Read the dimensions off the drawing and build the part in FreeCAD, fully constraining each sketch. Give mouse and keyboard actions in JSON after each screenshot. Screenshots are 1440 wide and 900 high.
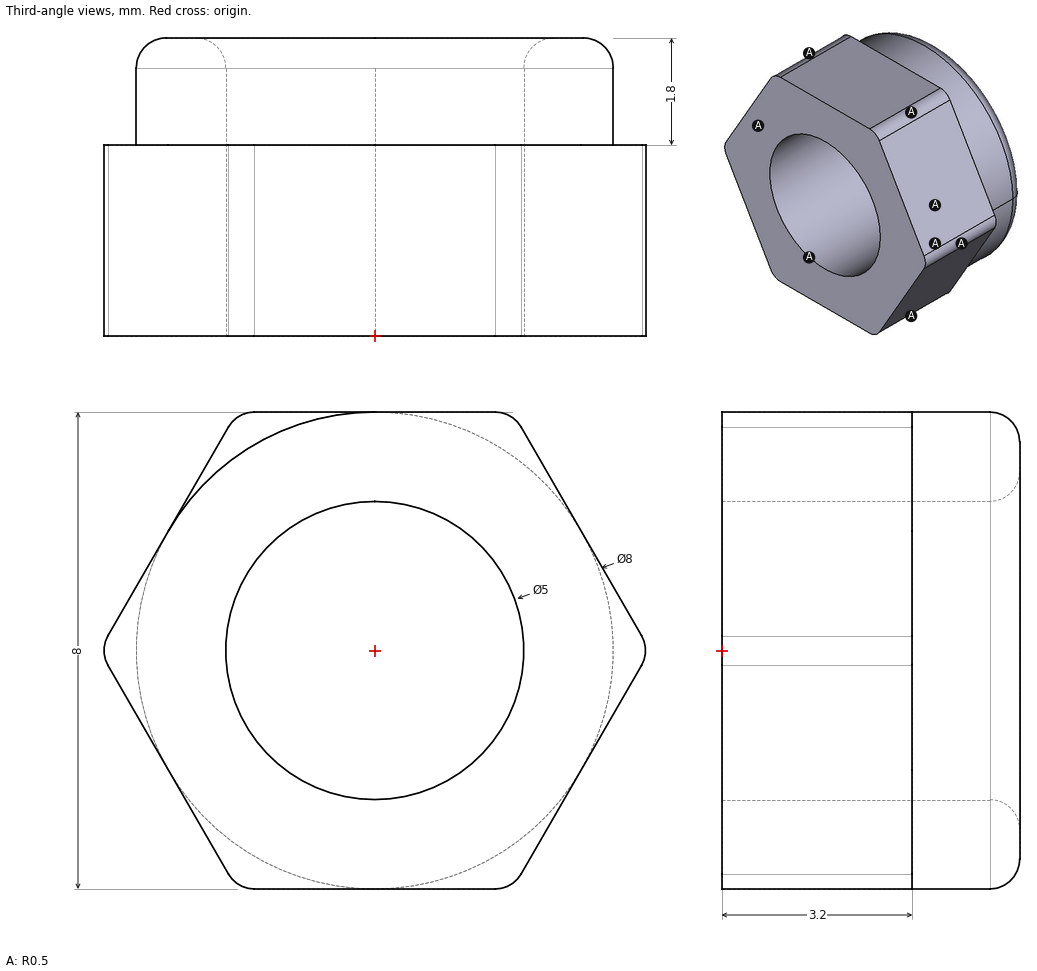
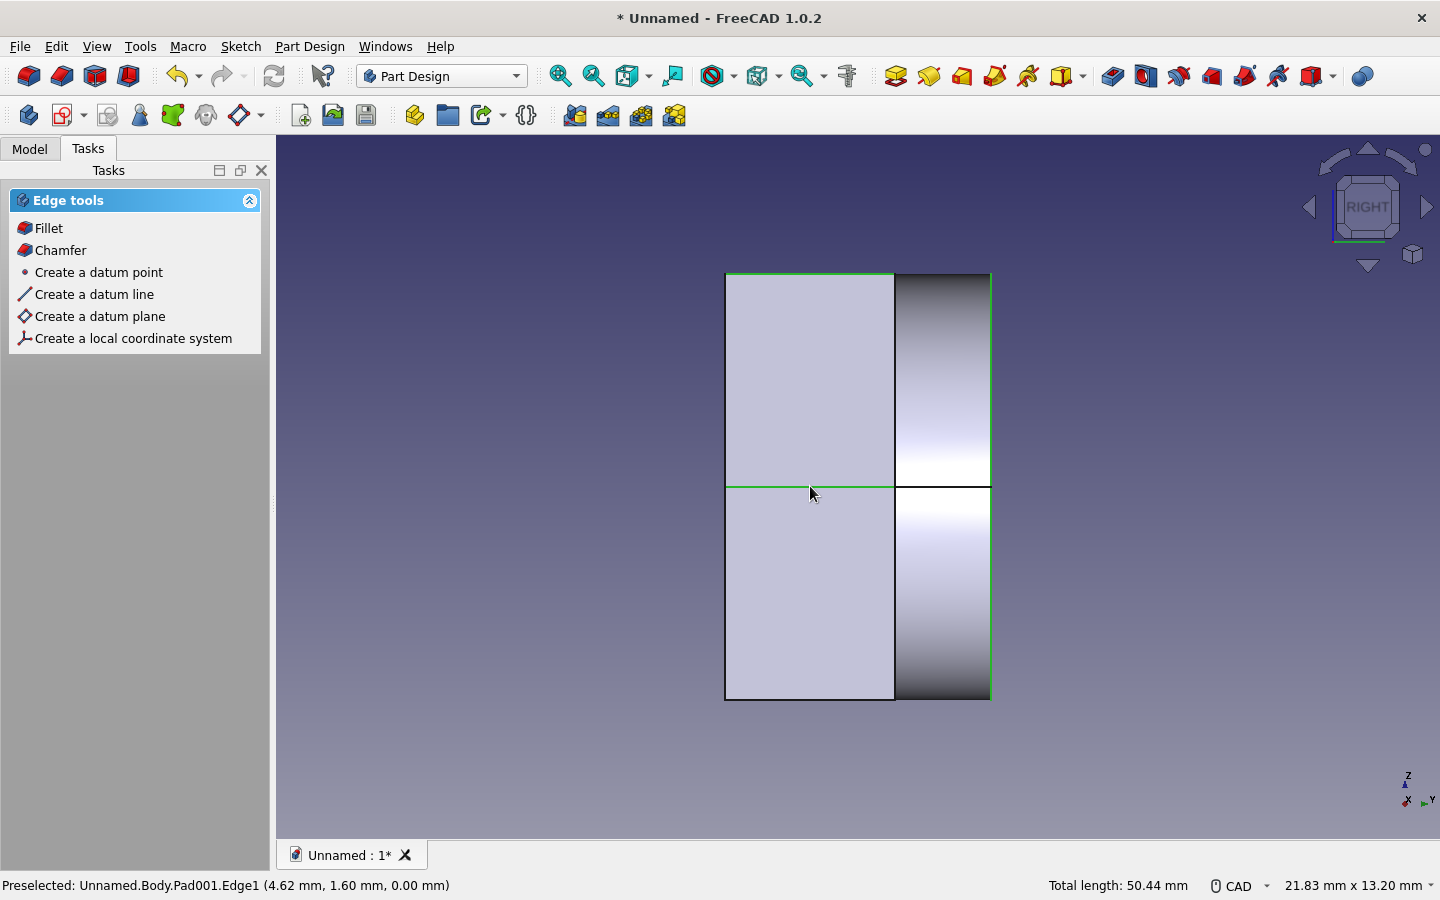
{"action": "key", "text": "5"}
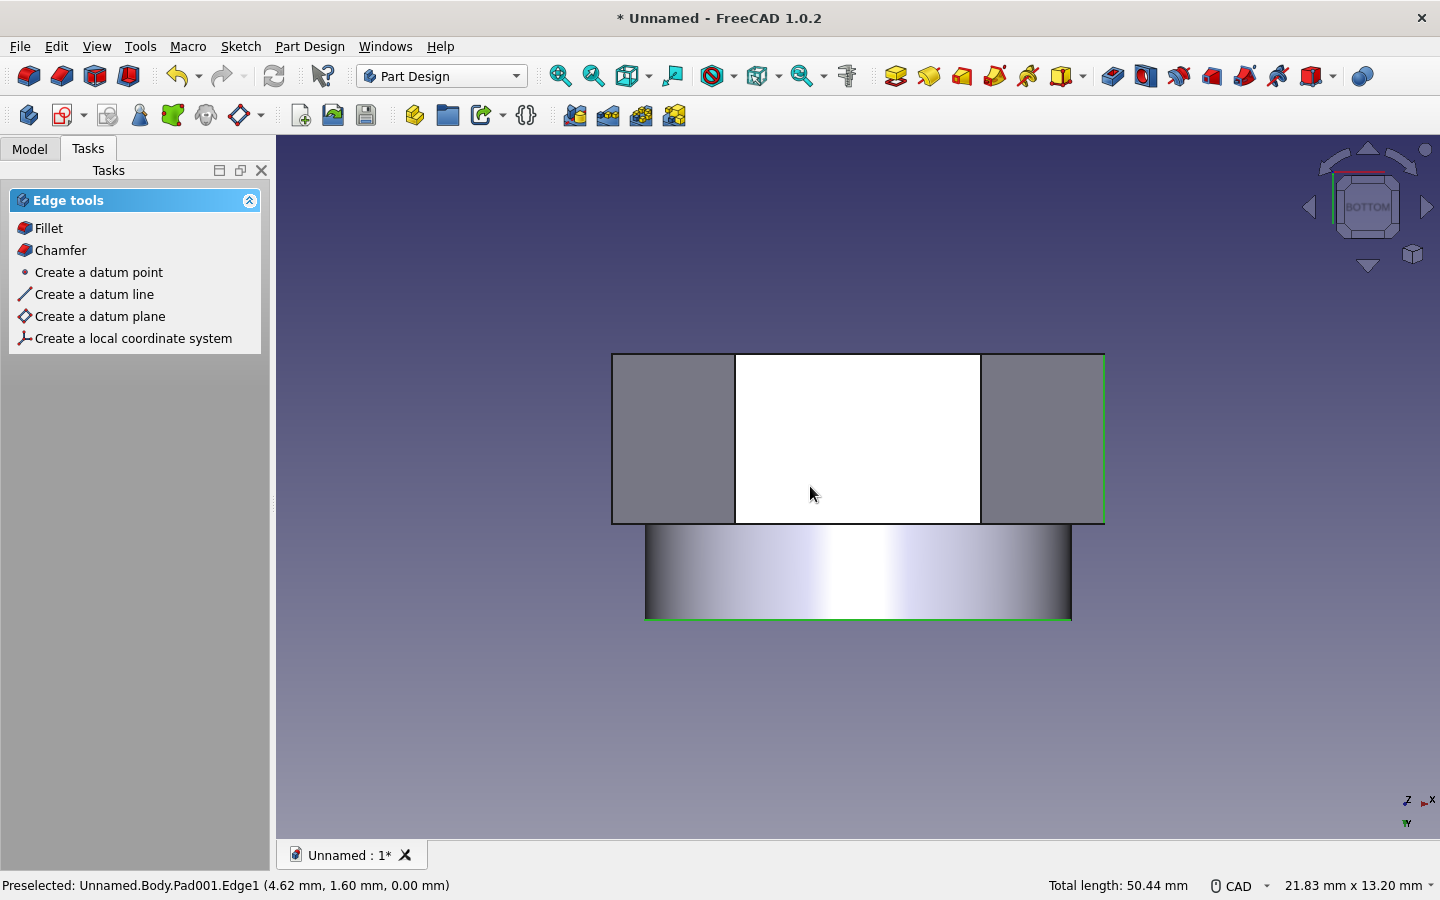
{"action": "left_click", "coordinate": [561, 76]}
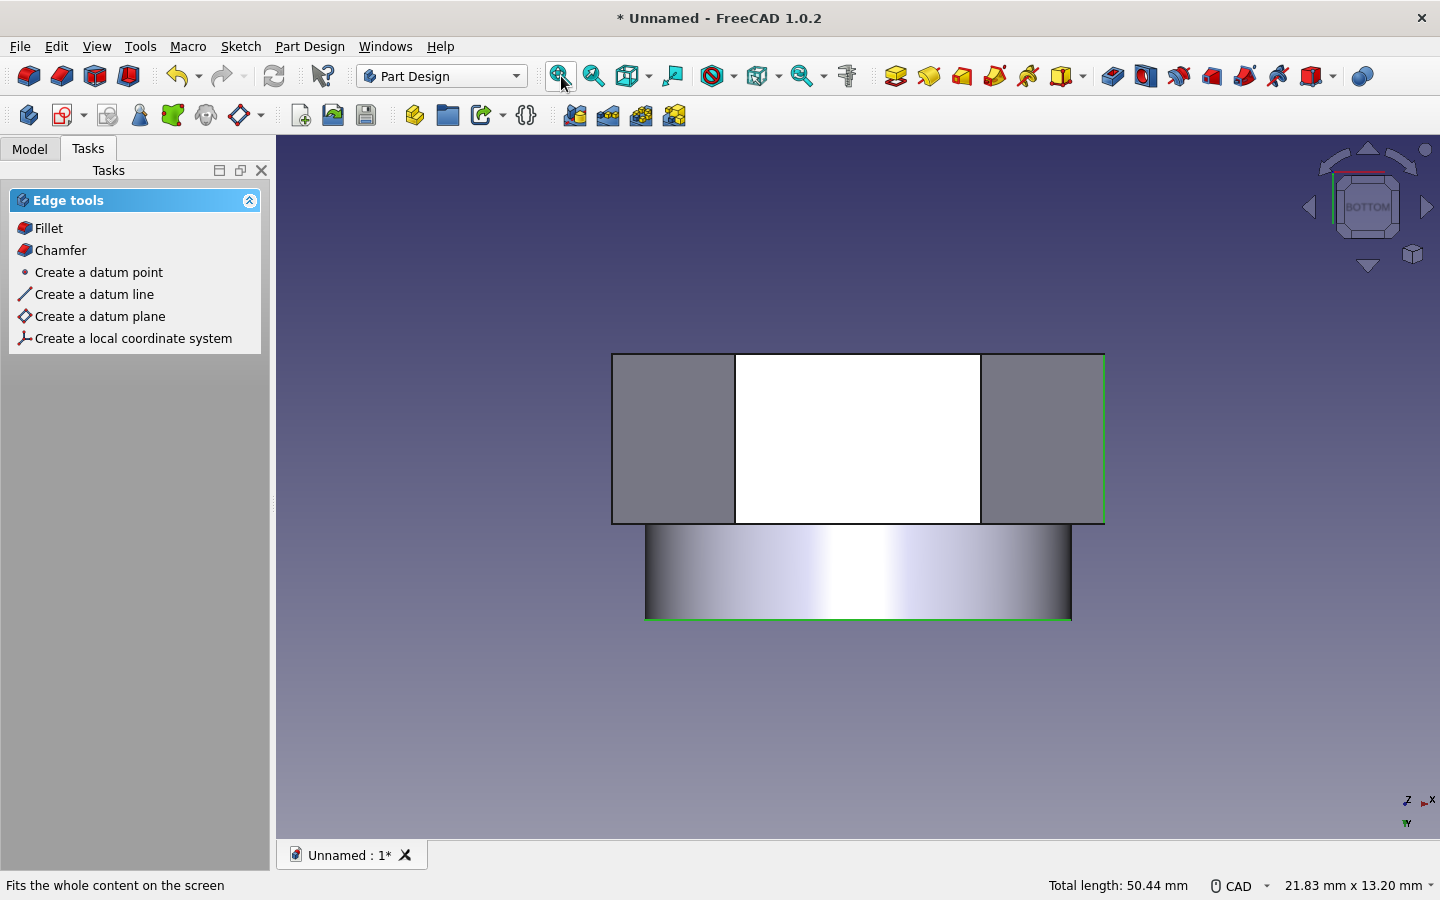
{"action": "left_click", "coordinate": [735, 438], "text": "ctrl"}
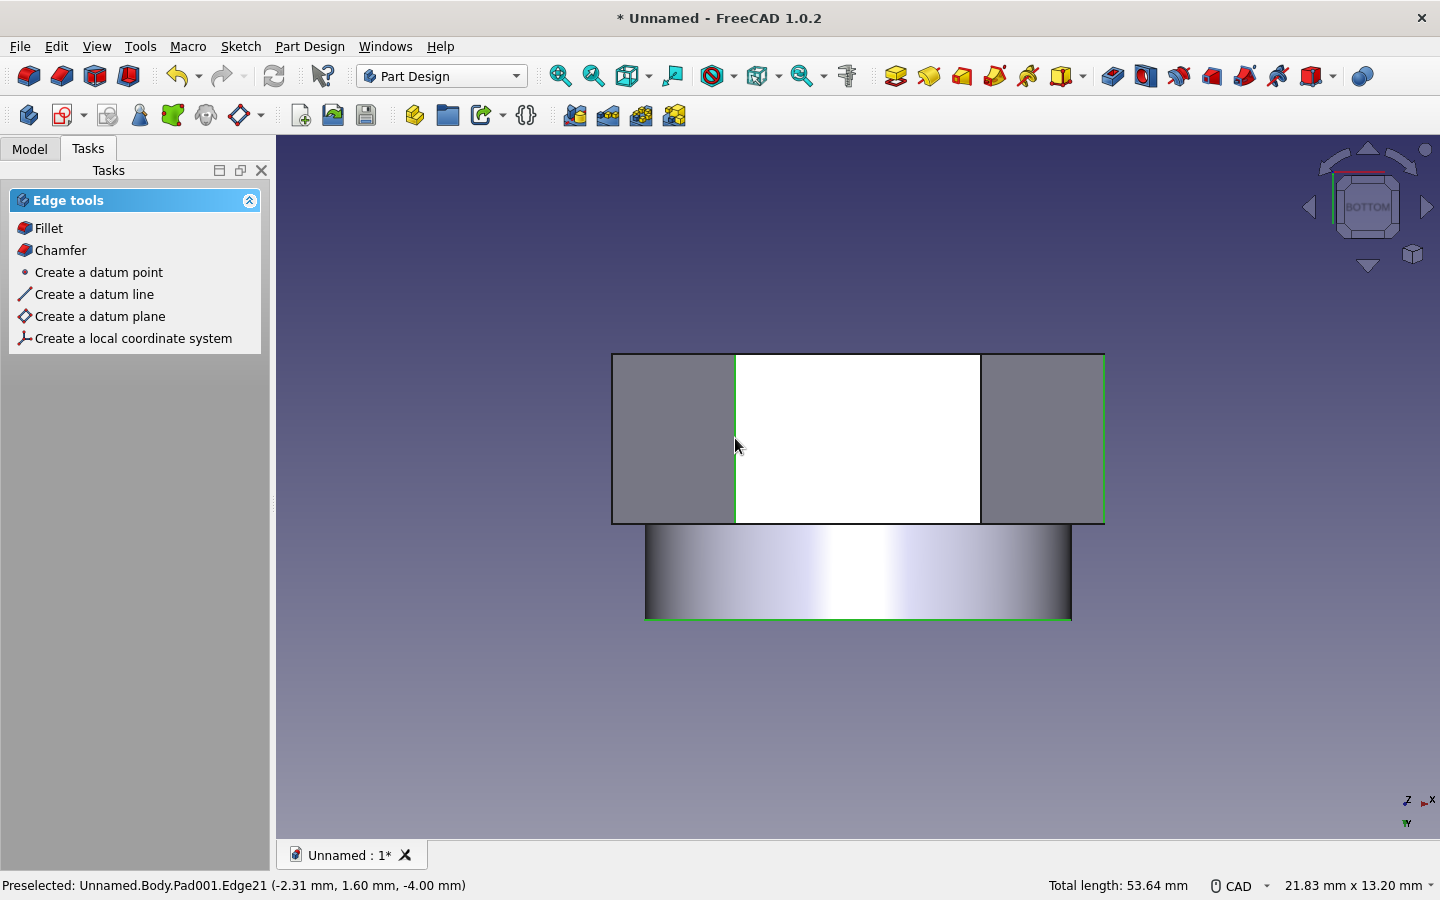
{"action": "left_click", "coordinate": [981, 438], "text": "ctrl"}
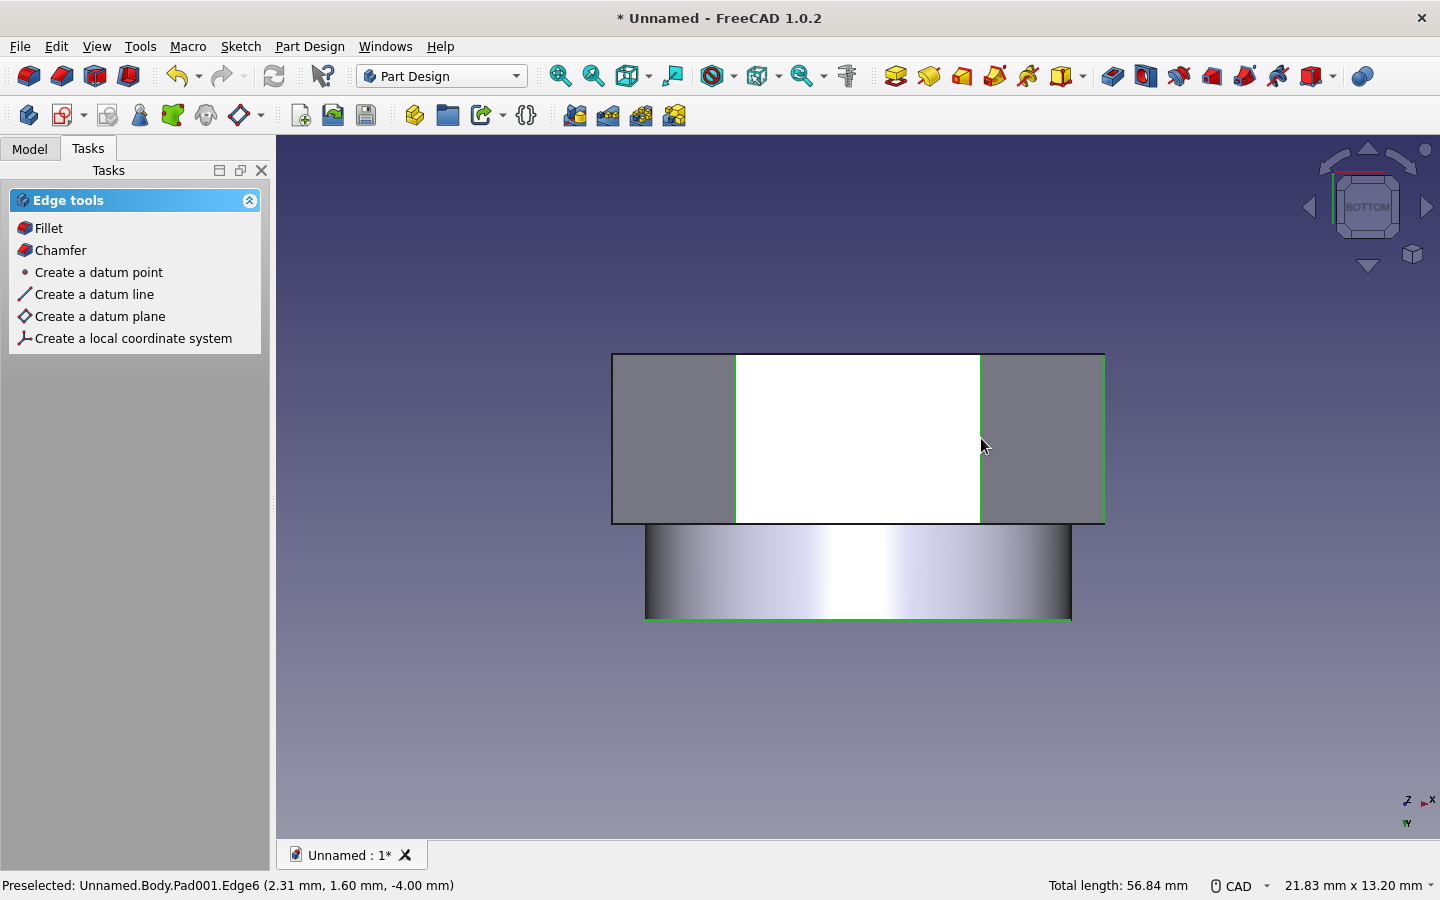
{"action": "key", "text": "4"}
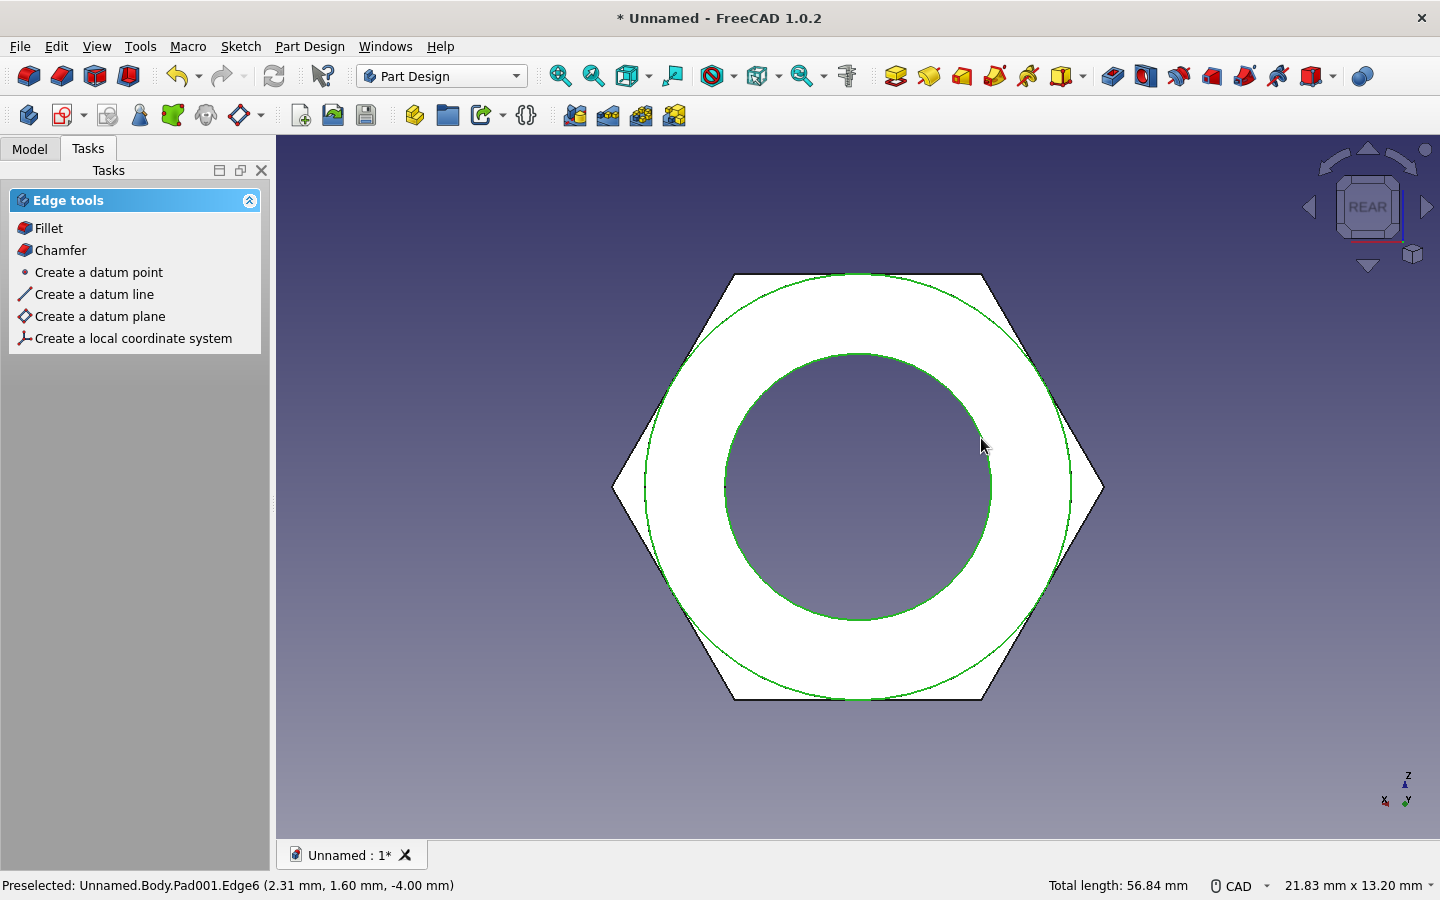
{"action": "key", "text": "6"}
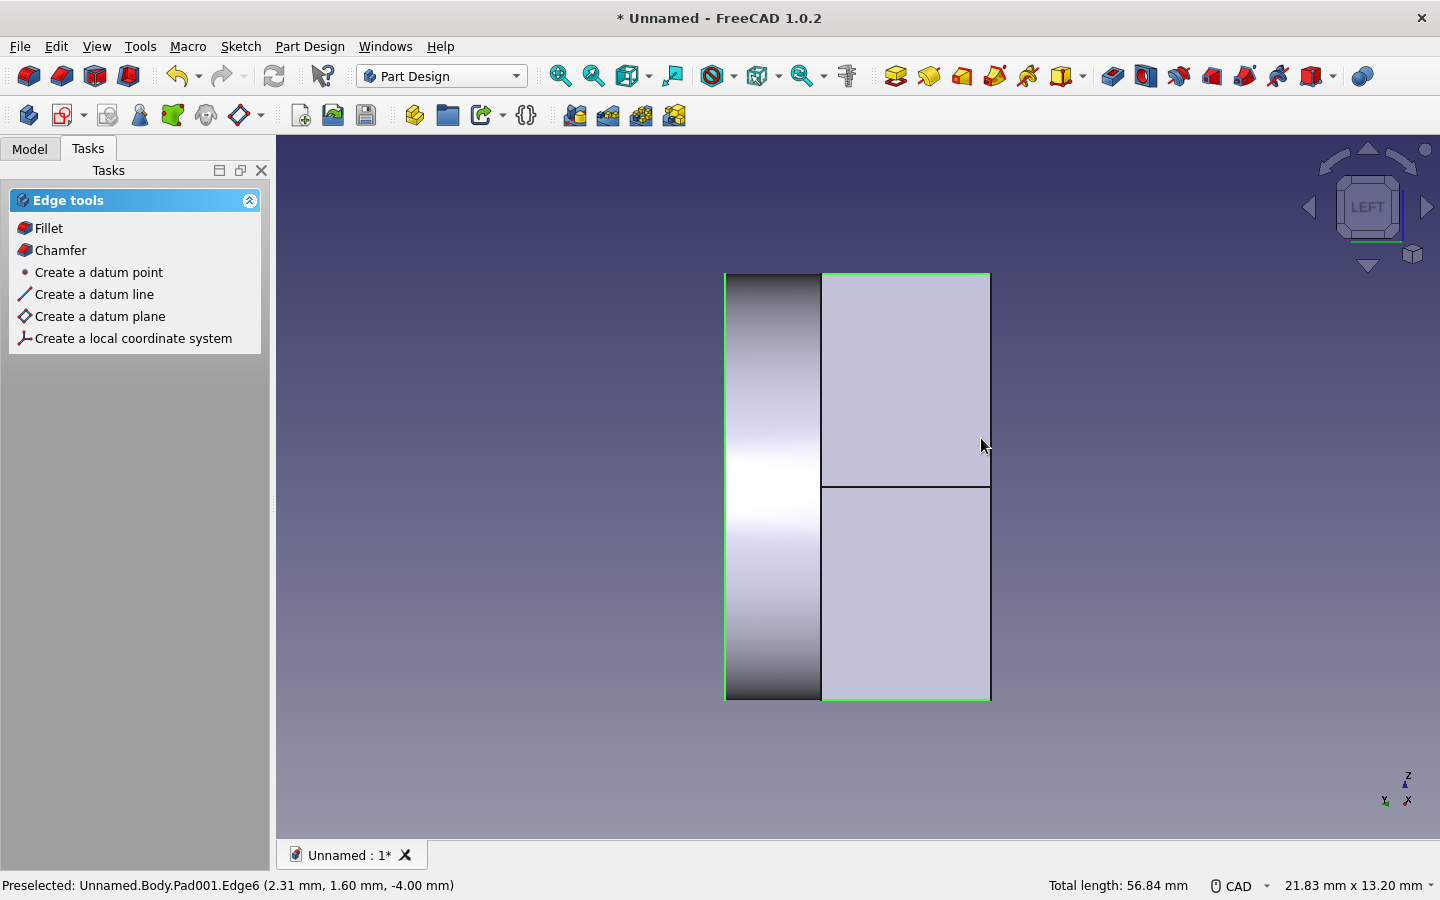
{"action": "left_click", "coordinate": [906, 486], "text": "ctrl"}